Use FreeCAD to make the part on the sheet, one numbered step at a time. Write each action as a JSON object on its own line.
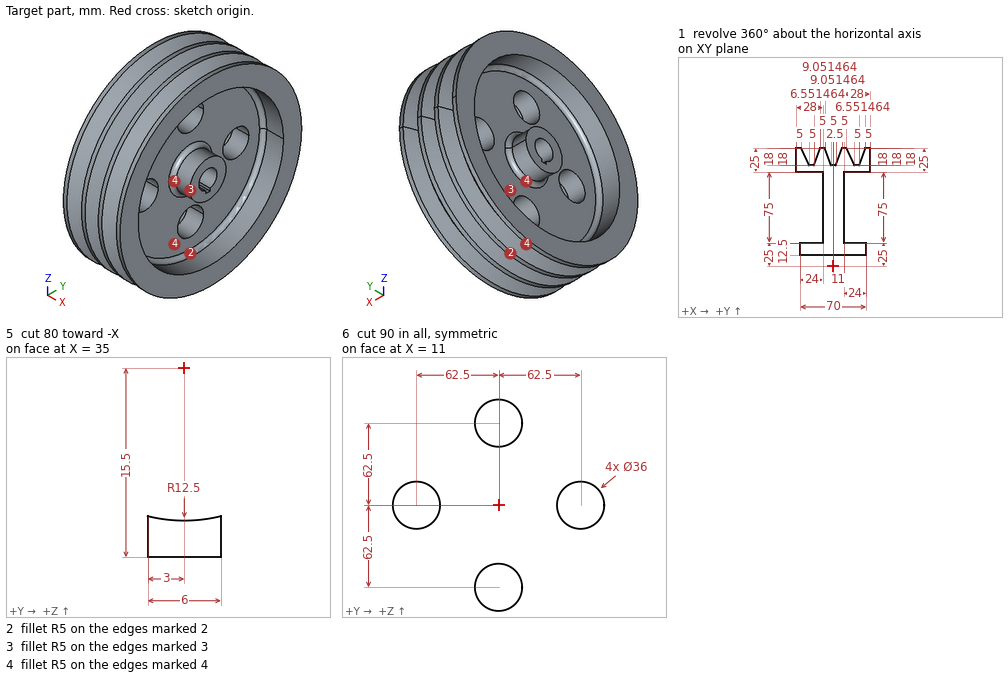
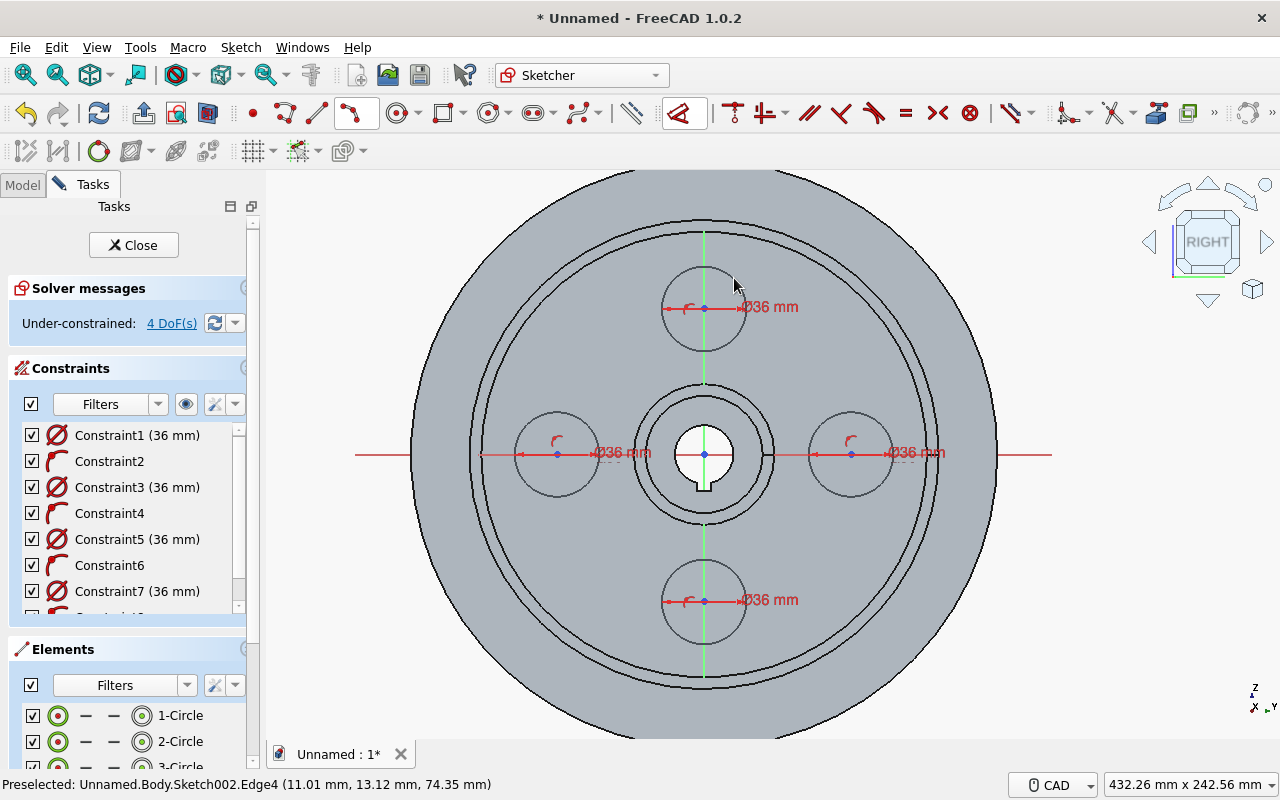
{"action": "left_click", "coordinate": [851, 454]}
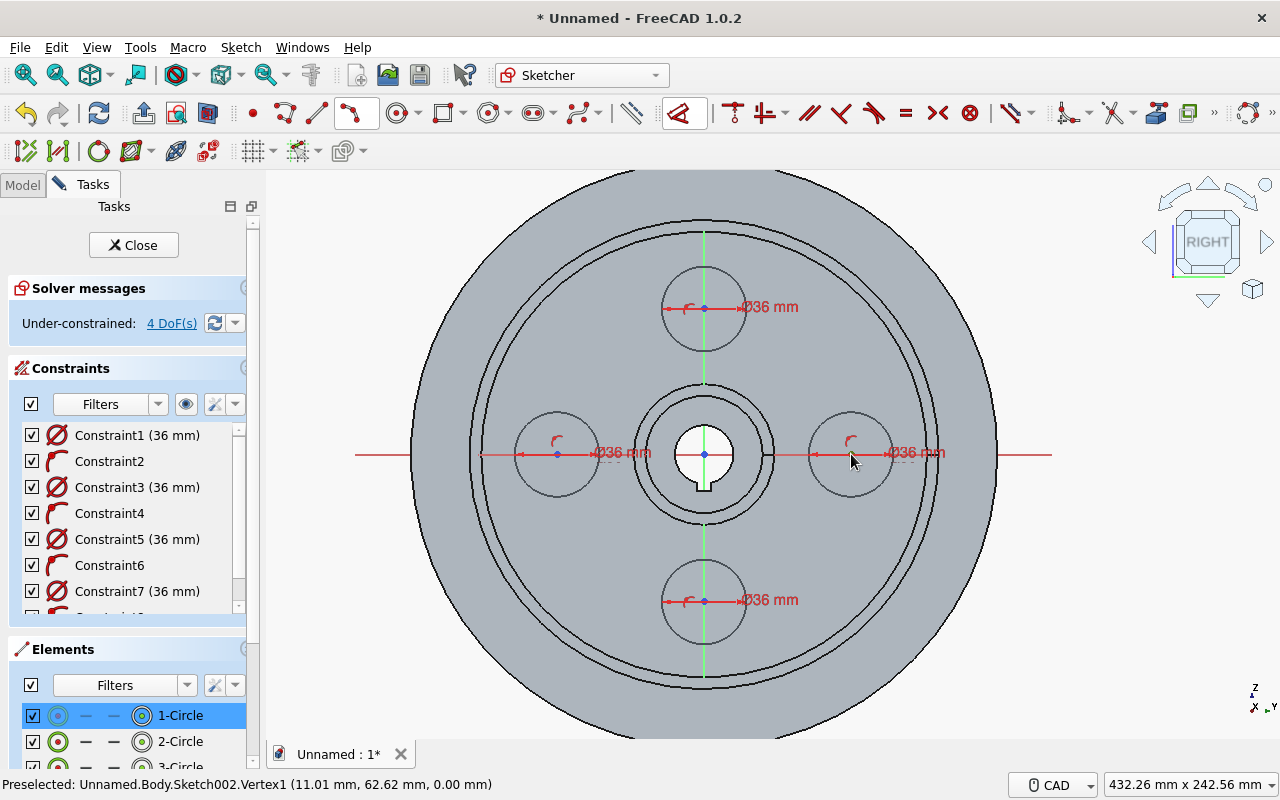
{"action": "key", "text": "l"}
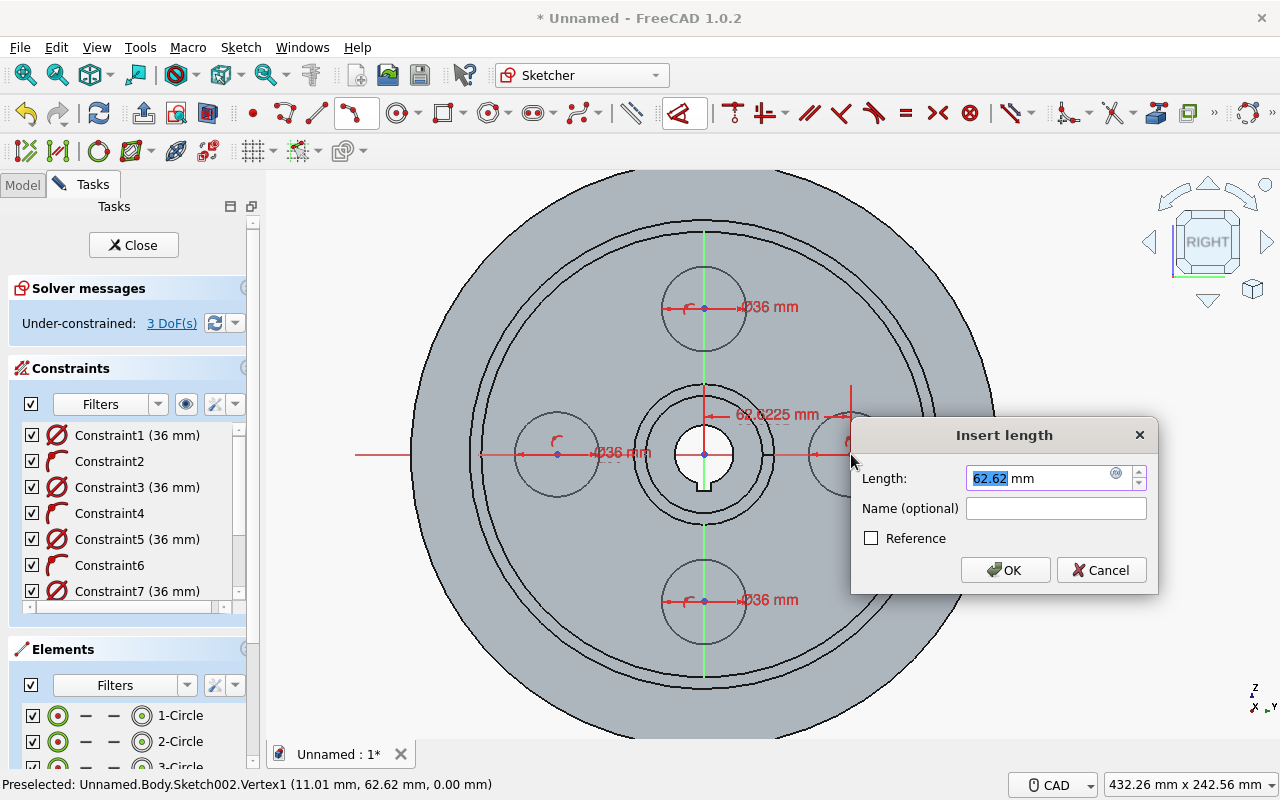
{"action": "type", "text": "62.5"}
{"action": "key", "text": "Return"}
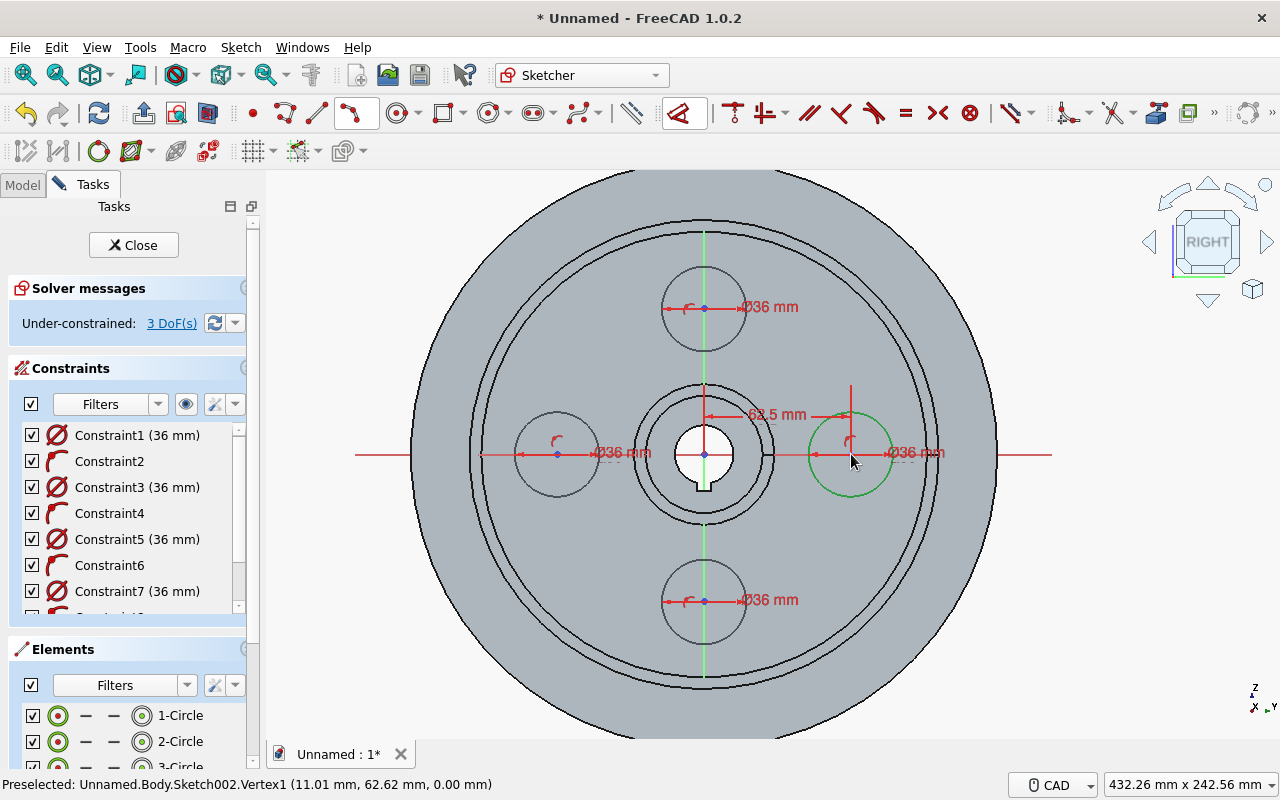
{"action": "left_click", "coordinate": [704, 602]}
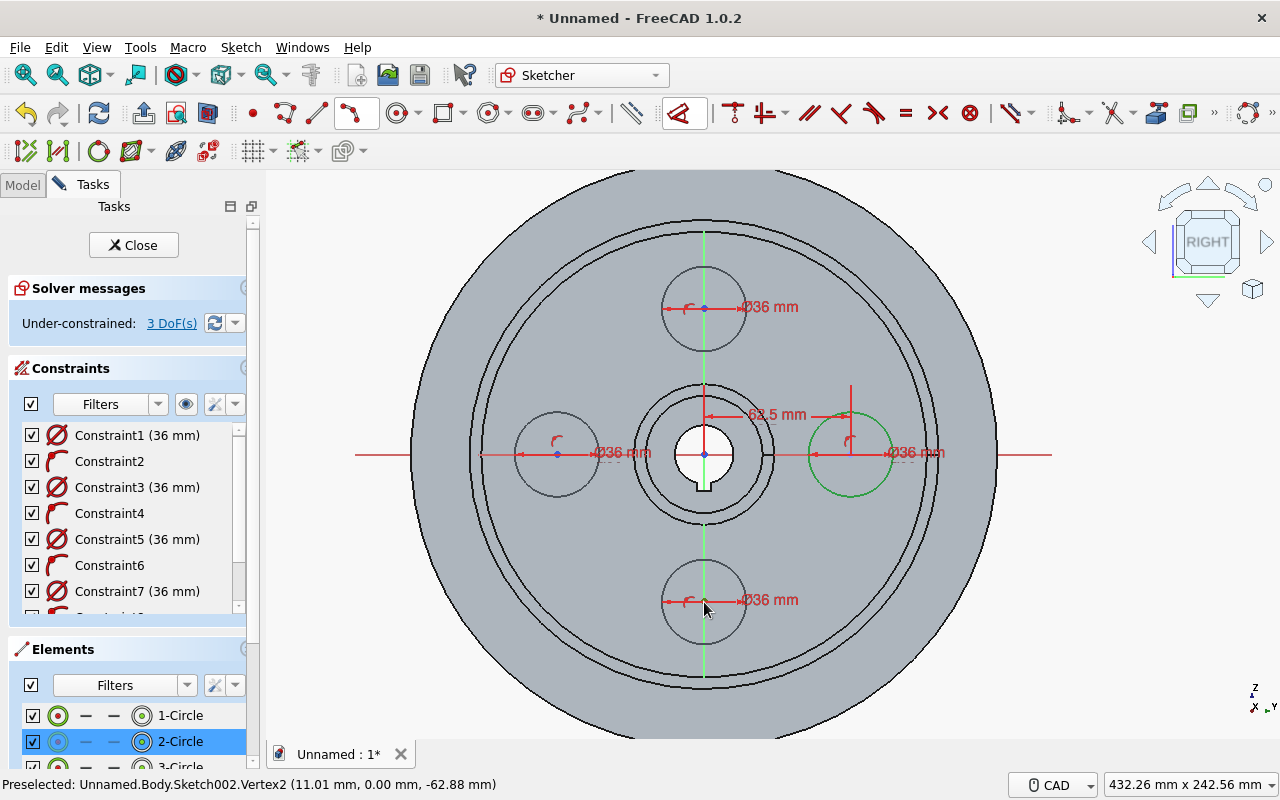
{"action": "key", "text": "i"}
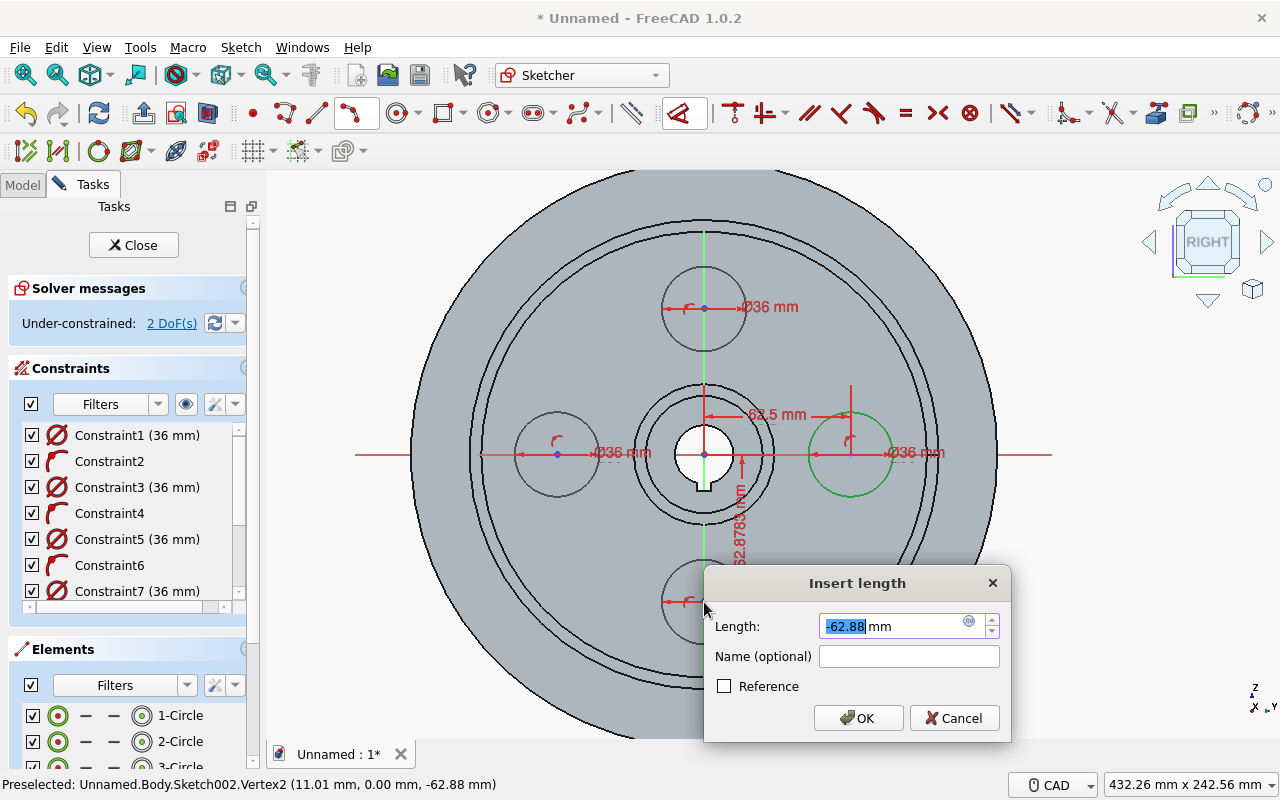
{"action": "type", "text": "-62.5"}
{"action": "key", "text": "Return"}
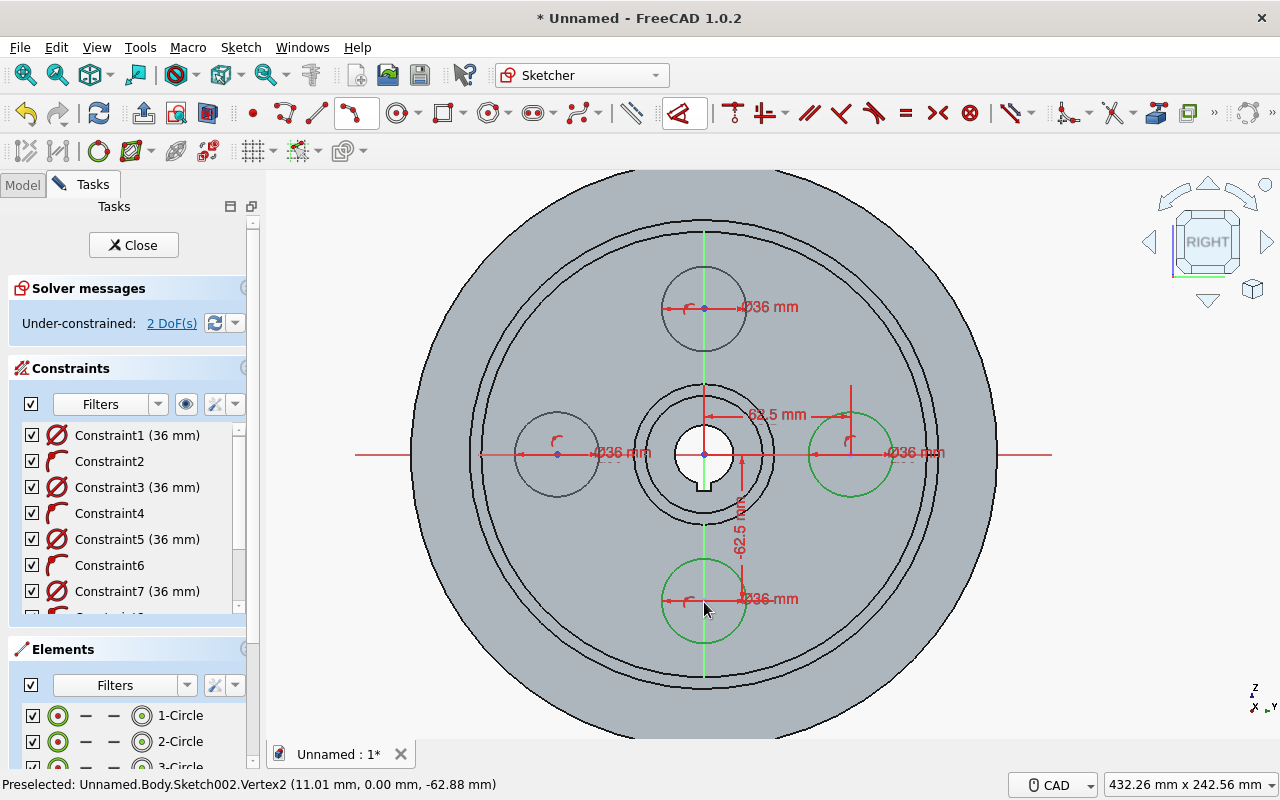
{"action": "left_click", "coordinate": [557, 454]}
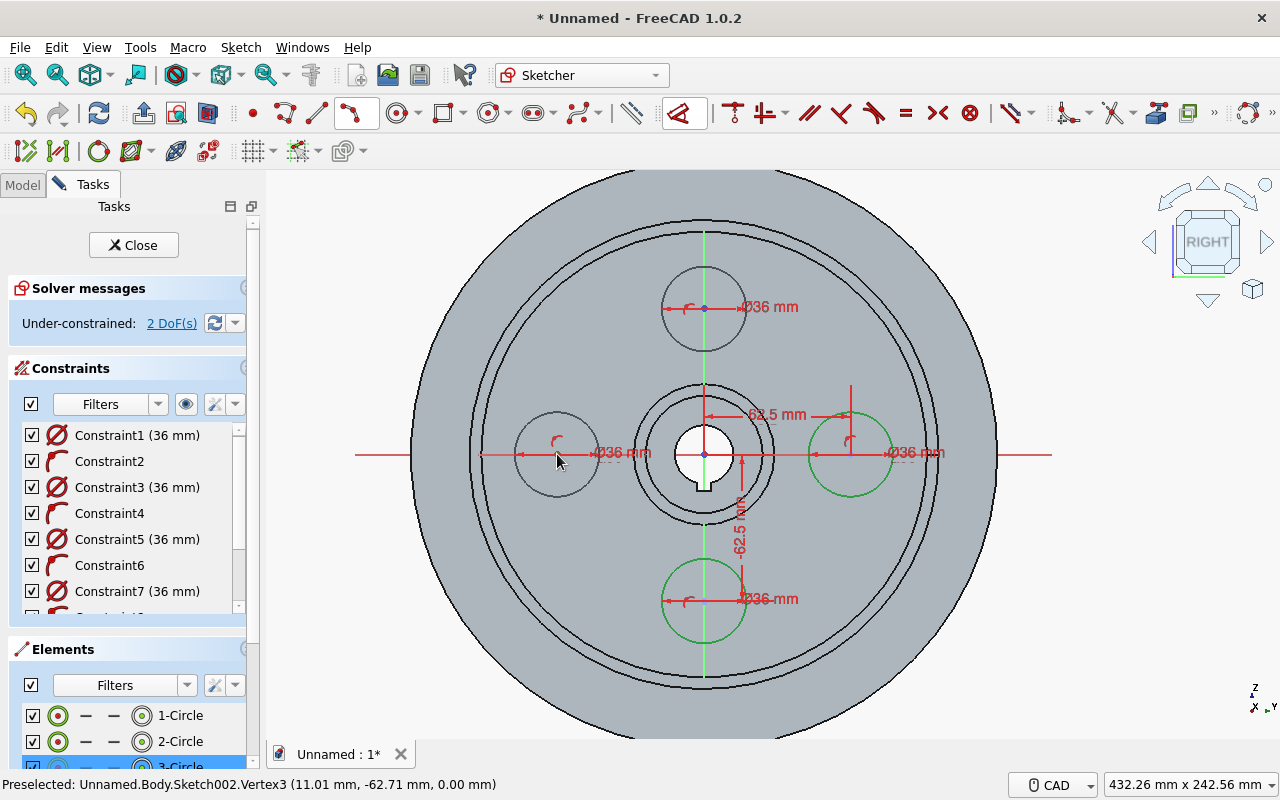
{"action": "key", "text": "l"}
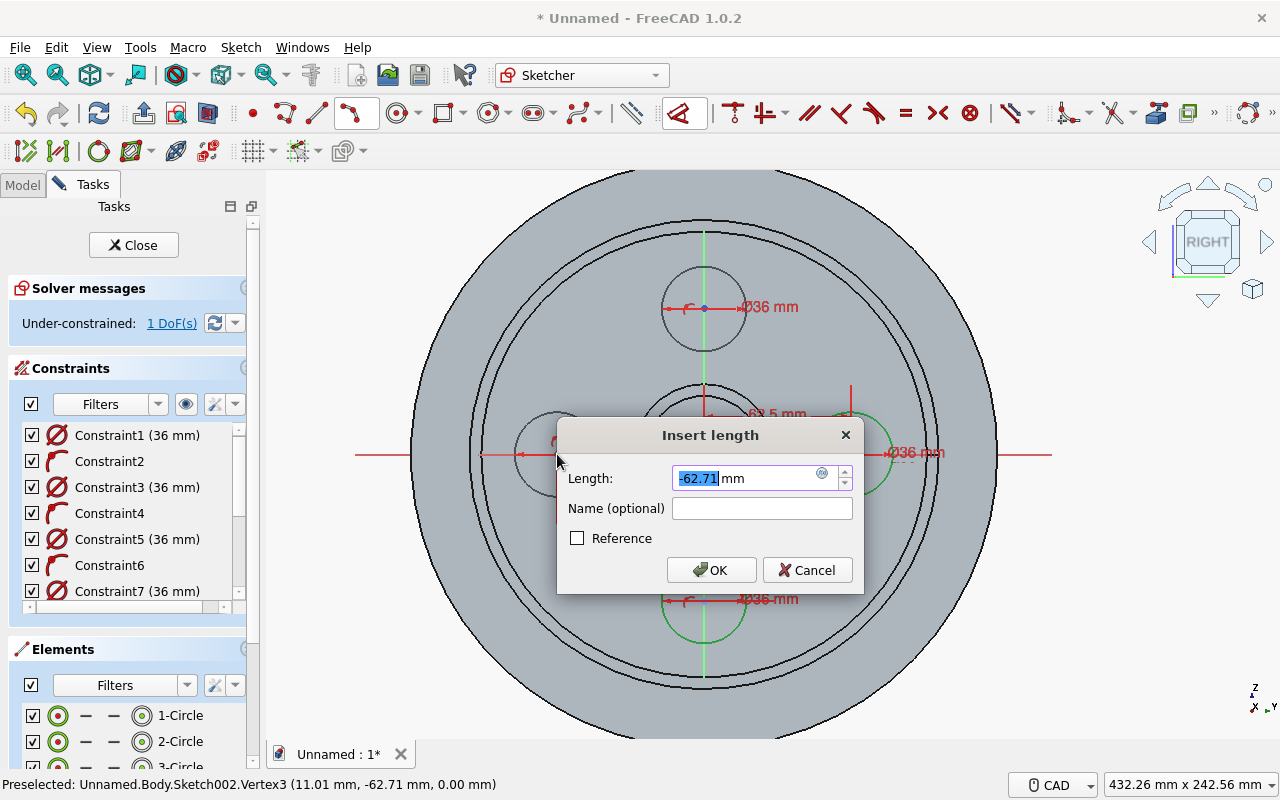
{"action": "type", "text": "-62.5"}
{"action": "key", "text": "Return"}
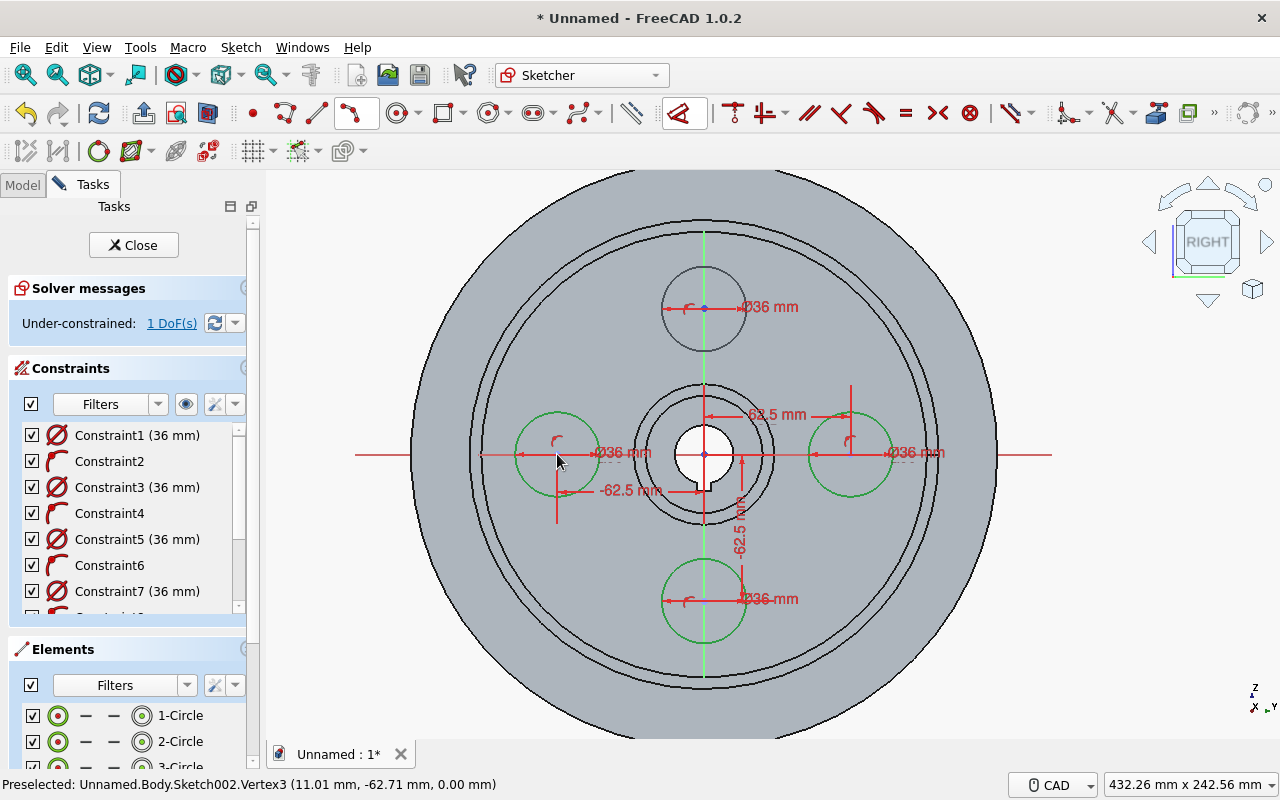
{"action": "left_click", "coordinate": [704, 309]}